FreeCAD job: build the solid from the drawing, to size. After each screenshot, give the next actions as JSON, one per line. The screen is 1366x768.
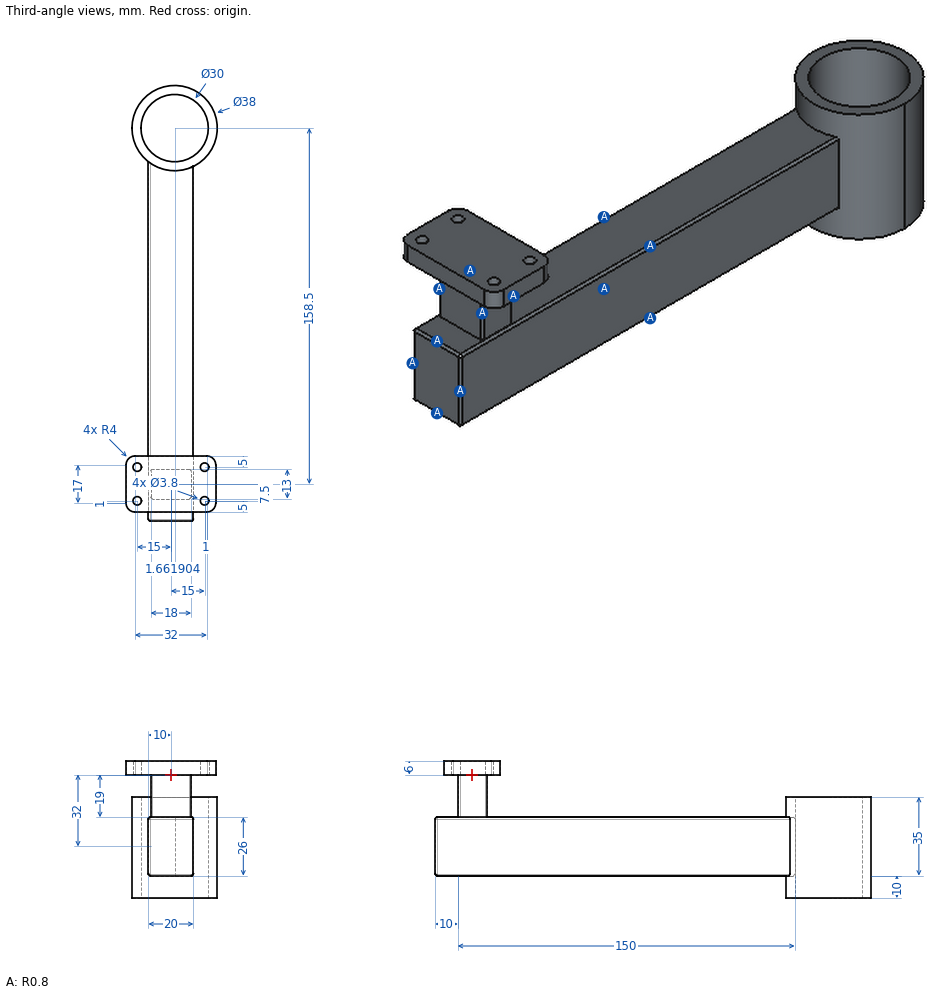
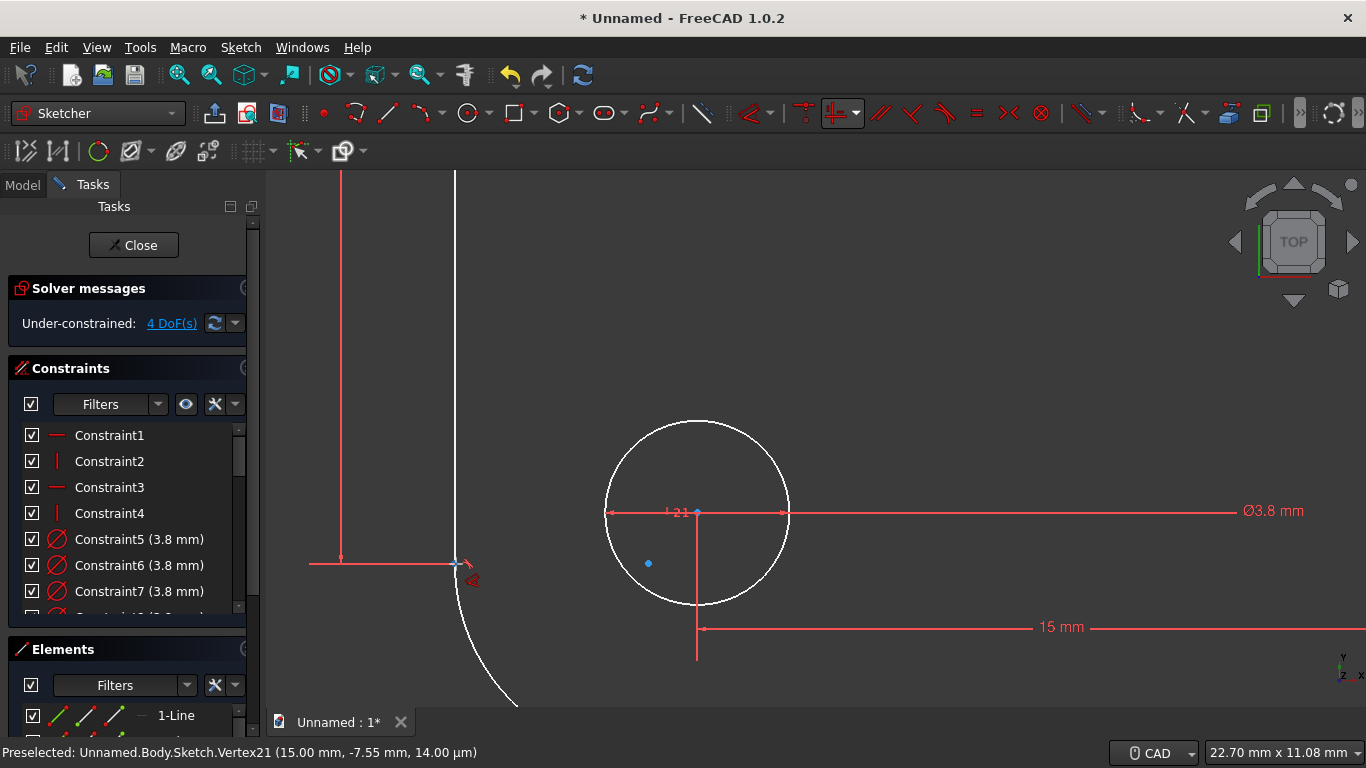
{"action": "left_click", "coordinate": [455, 564]}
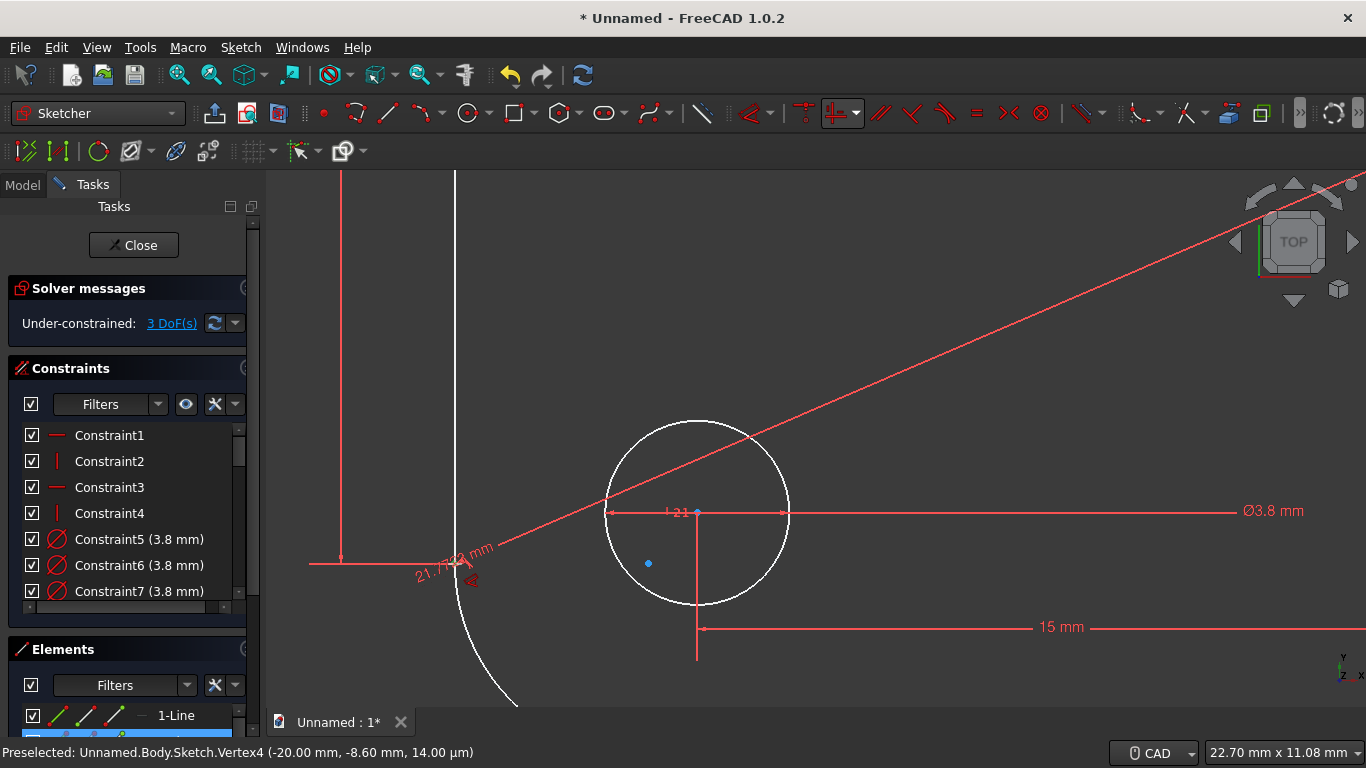
{"action": "left_click", "coordinate": [697, 513]}
{"action": "left_click", "coordinate": [421, 538]}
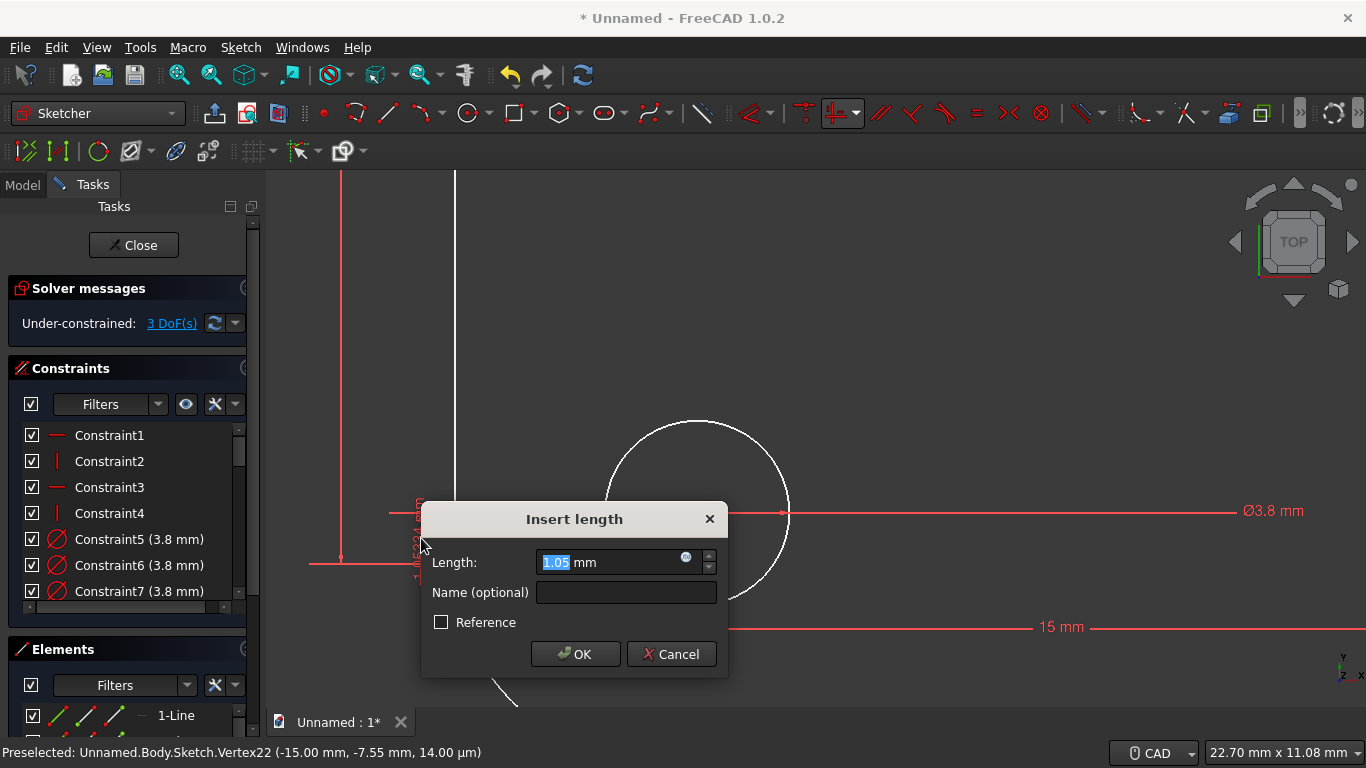
{"action": "type", "text": "1"}
{"action": "key", "text": "Return"}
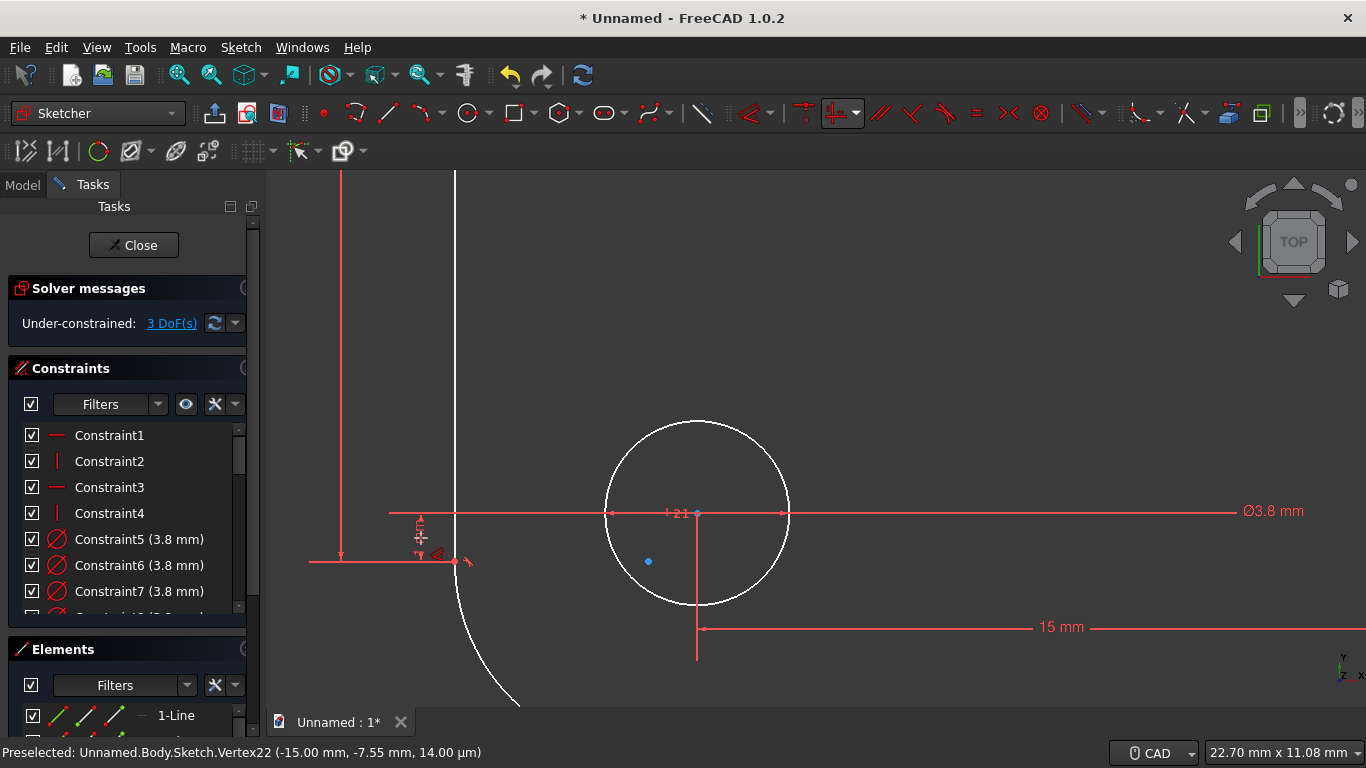
{"action": "scroll", "coordinate": [456, 564], "scroll_direction": "down", "scroll_amount": 6}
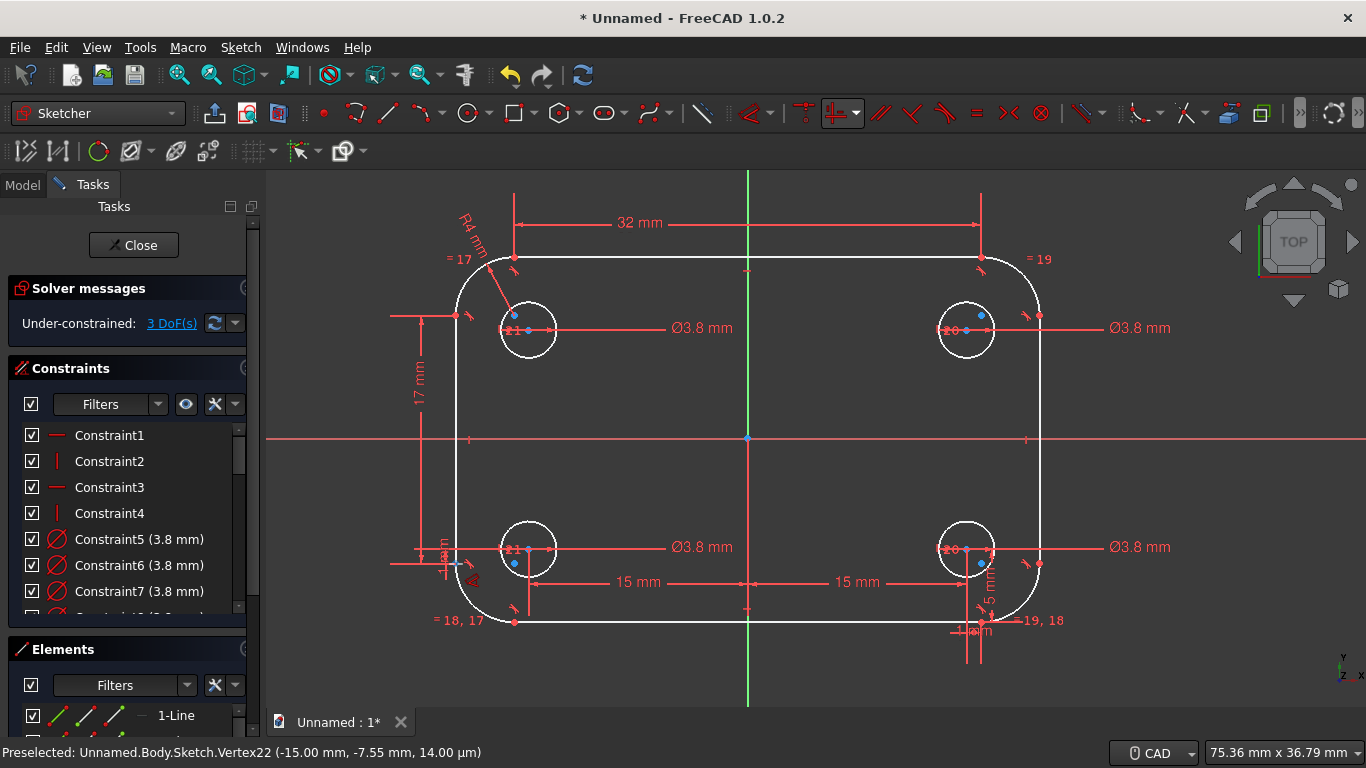
{"action": "left_click", "coordinate": [981, 257]}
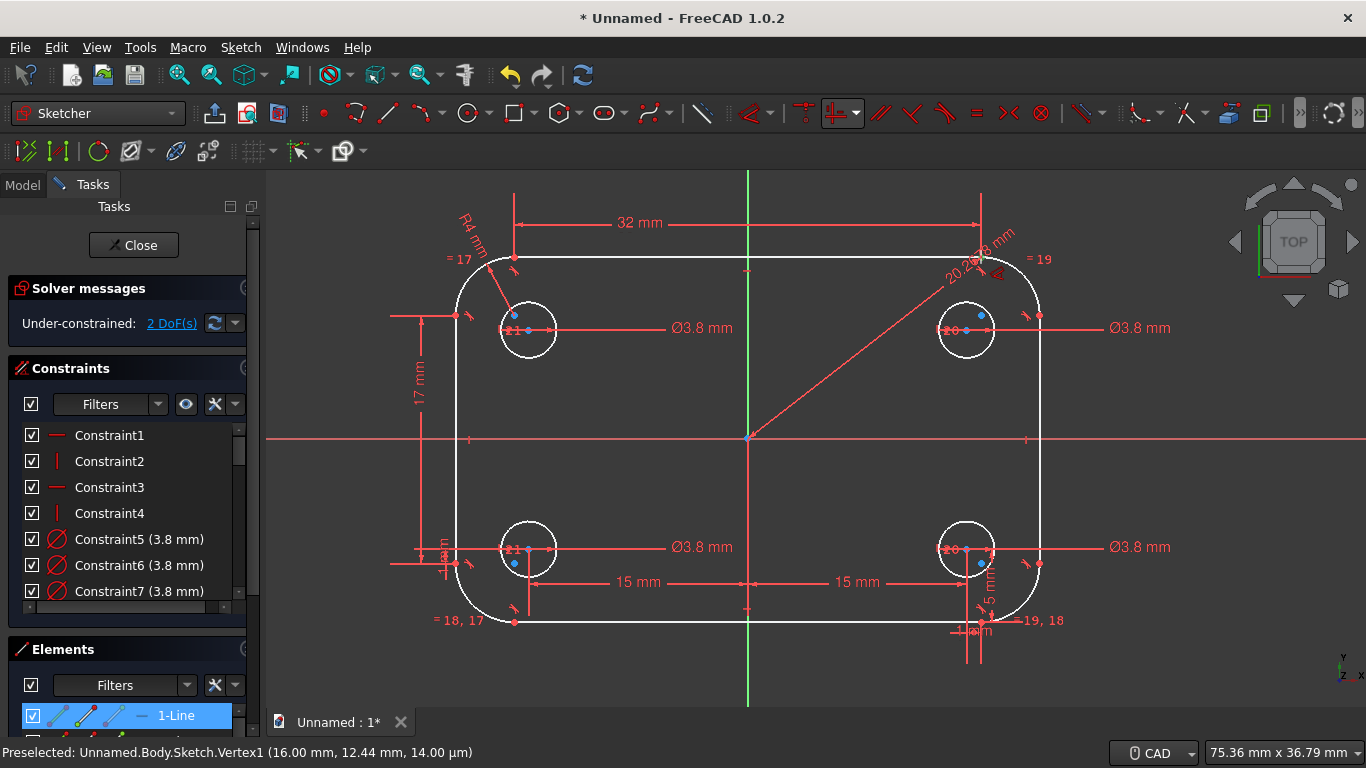
{"action": "left_click", "coordinate": [967, 330]}
{"action": "left_click", "coordinate": [1015, 294]}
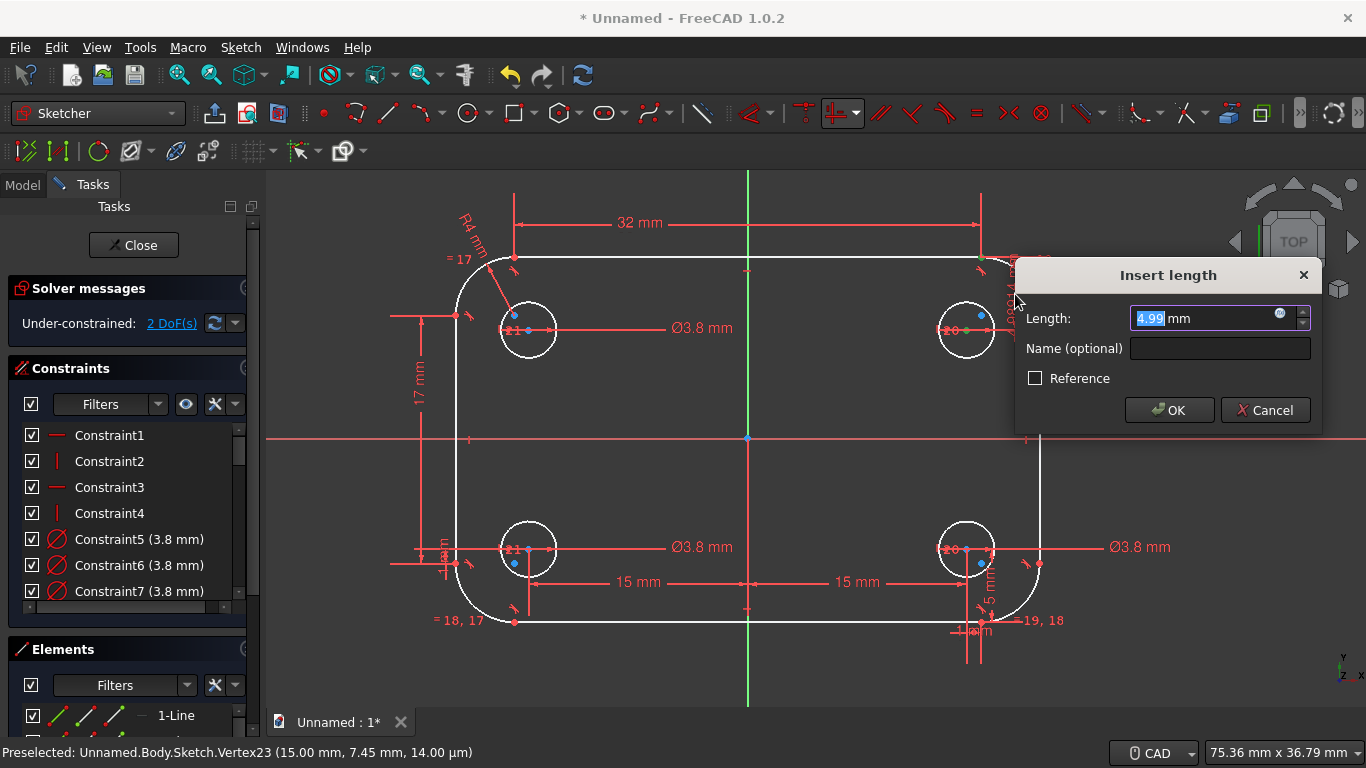
{"action": "type", "text": "5"}
{"action": "key", "text": "Return"}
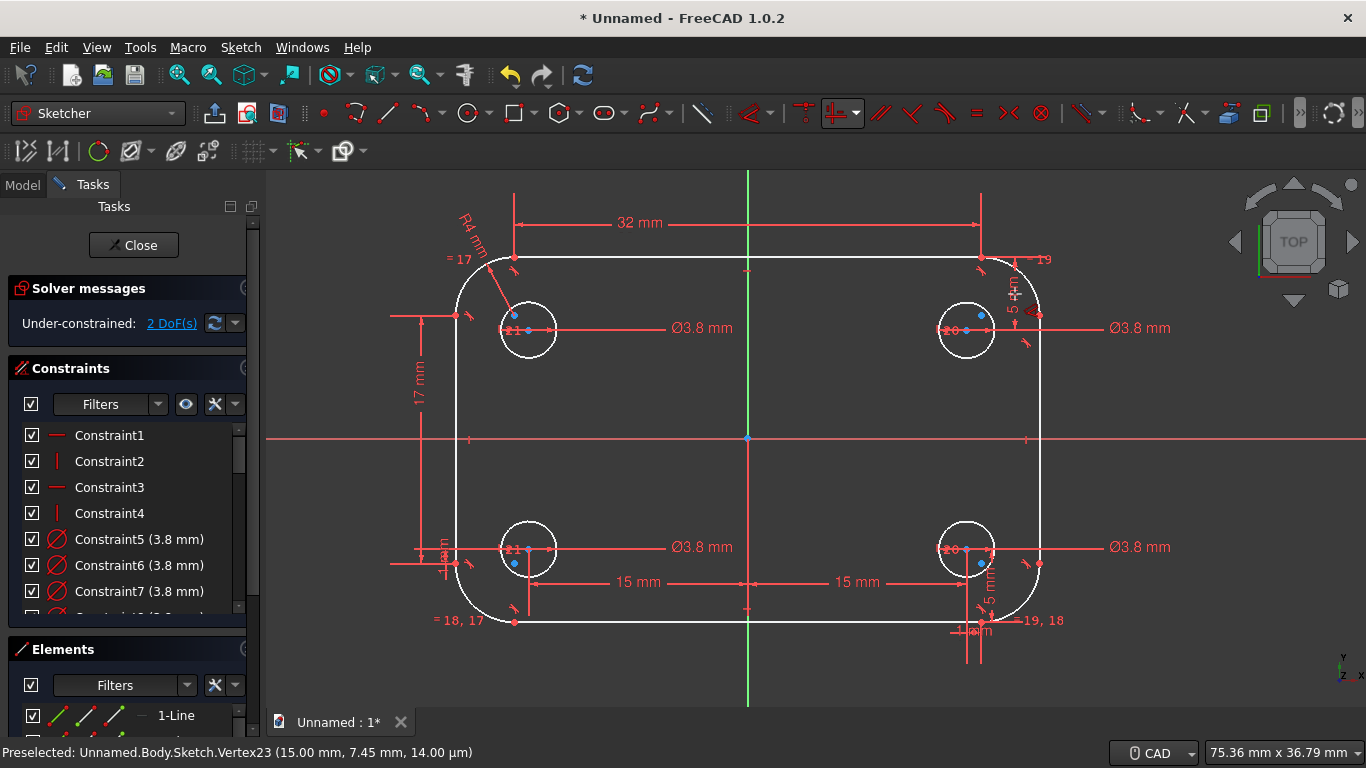
{"action": "left_click", "coordinate": [514, 257]}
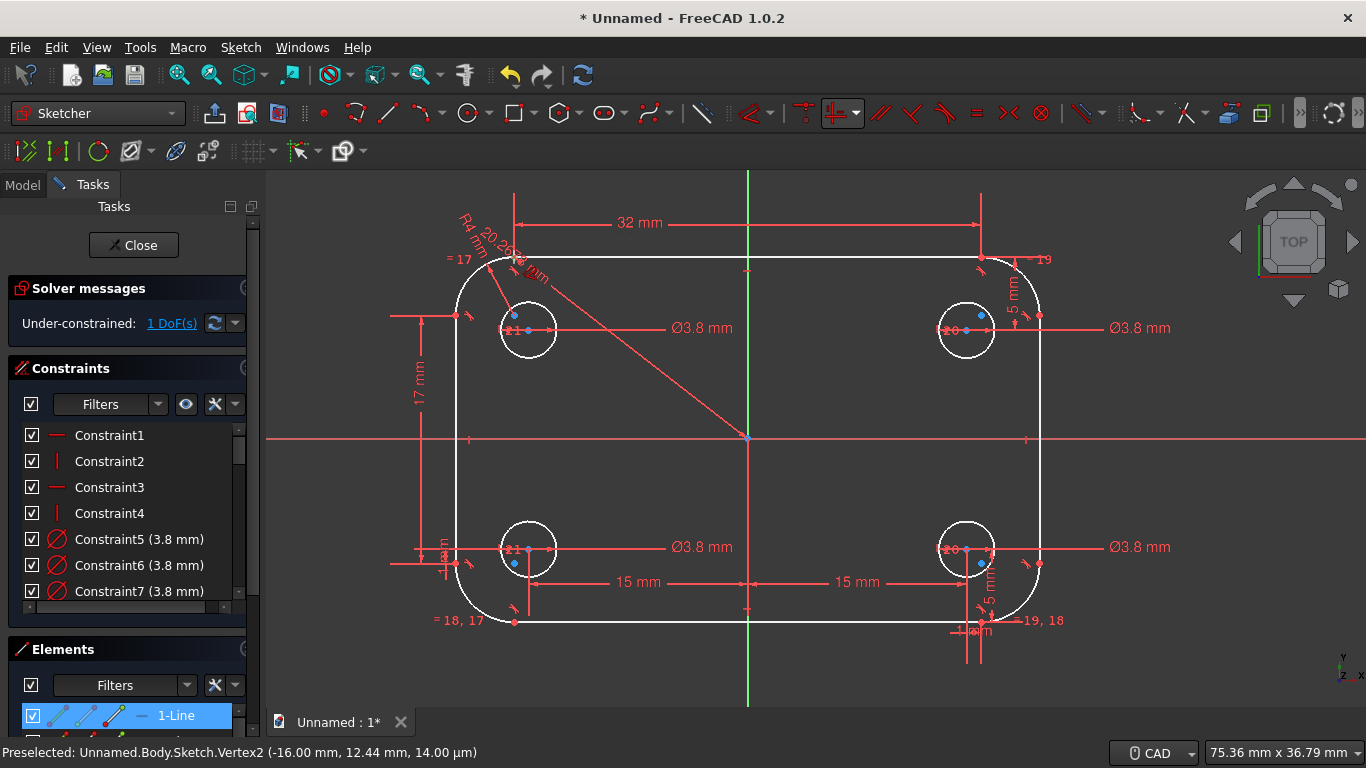
{"action": "left_click", "coordinate": [529, 330]}
{"action": "left_click", "coordinate": [480, 294]}